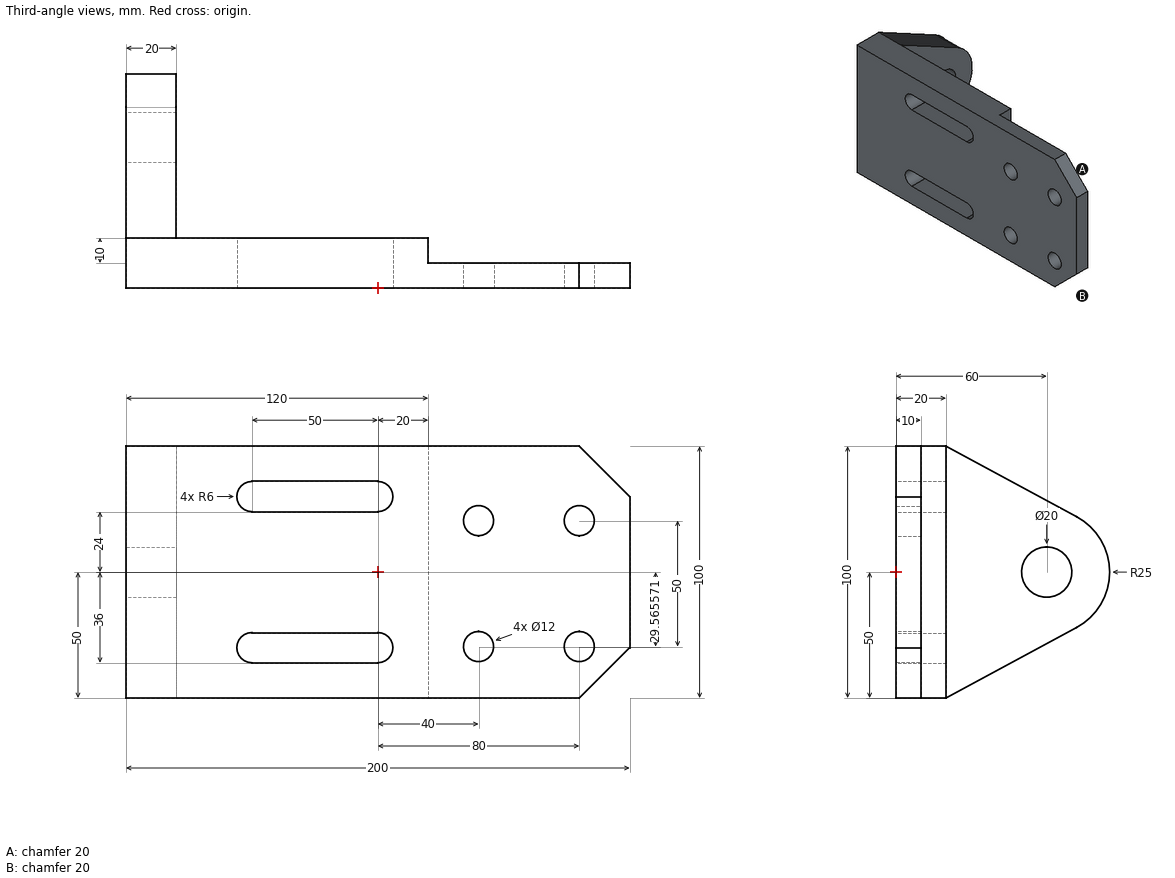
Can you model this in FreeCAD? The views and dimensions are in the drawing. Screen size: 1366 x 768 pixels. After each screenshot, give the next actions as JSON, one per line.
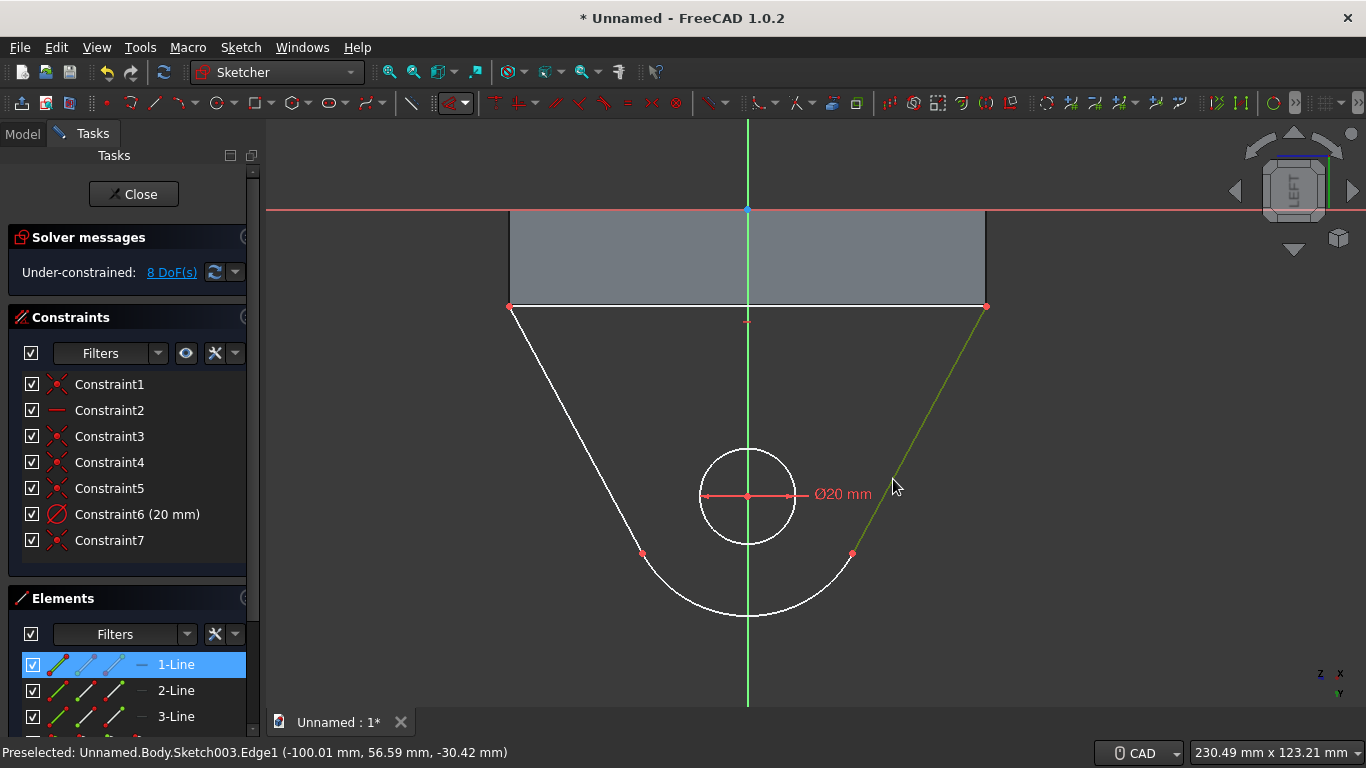
{"action": "left_click", "coordinate": [698, 605]}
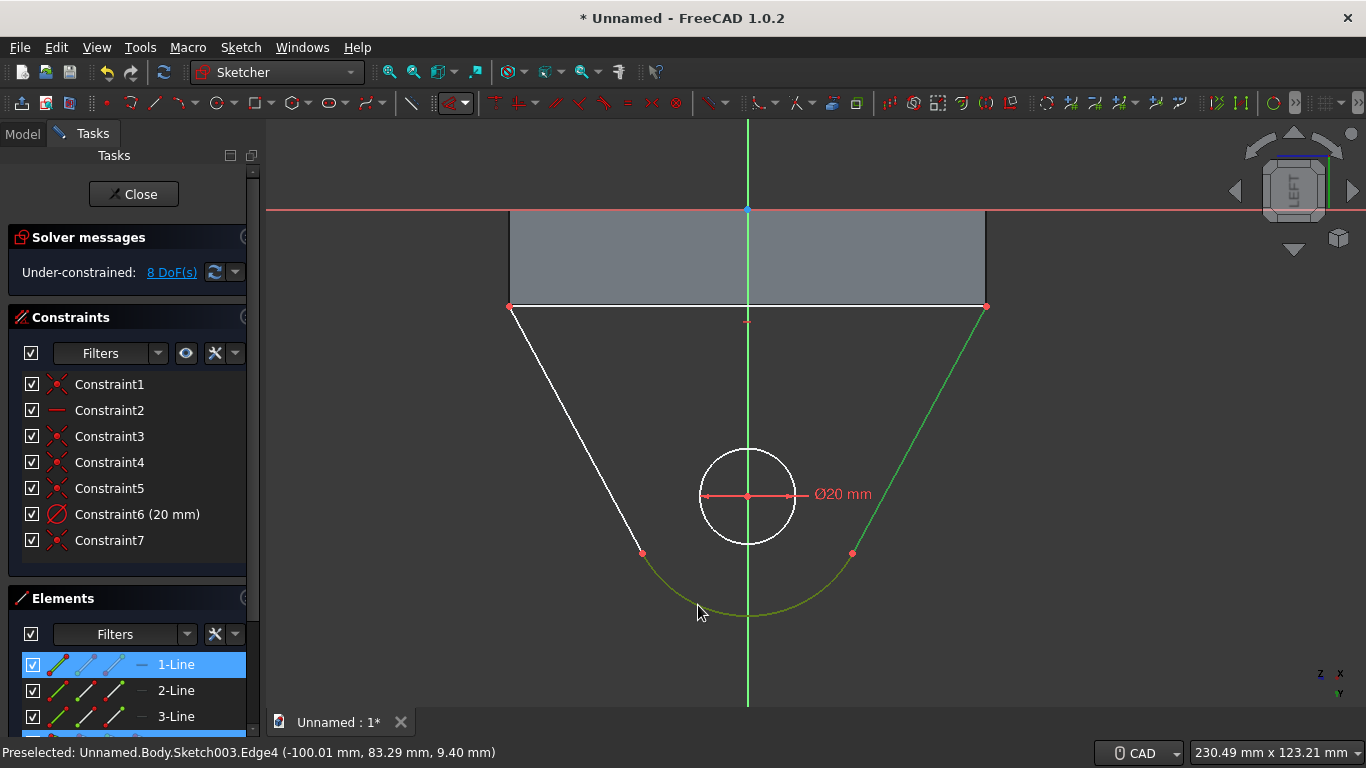
{"action": "left_click", "coordinate": [604, 104]}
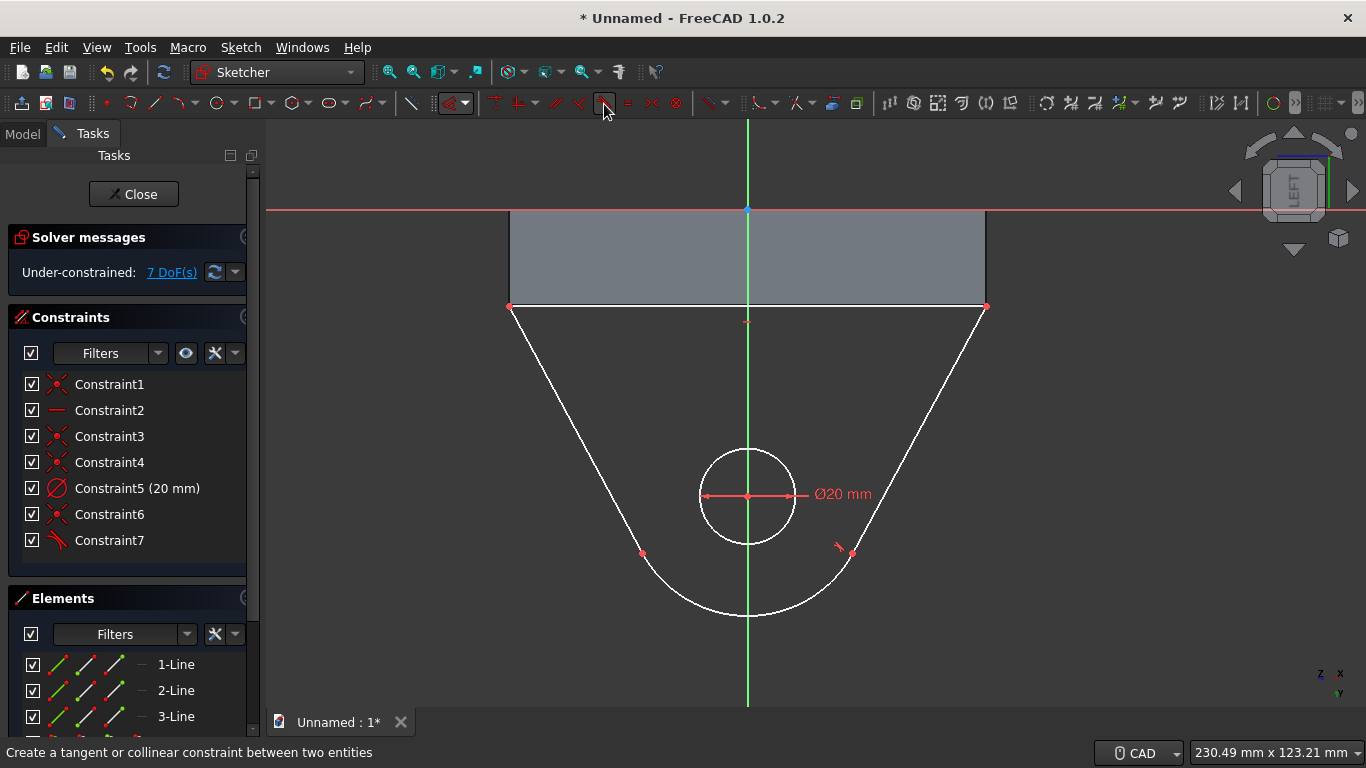
{"action": "left_click", "coordinate": [549, 381]}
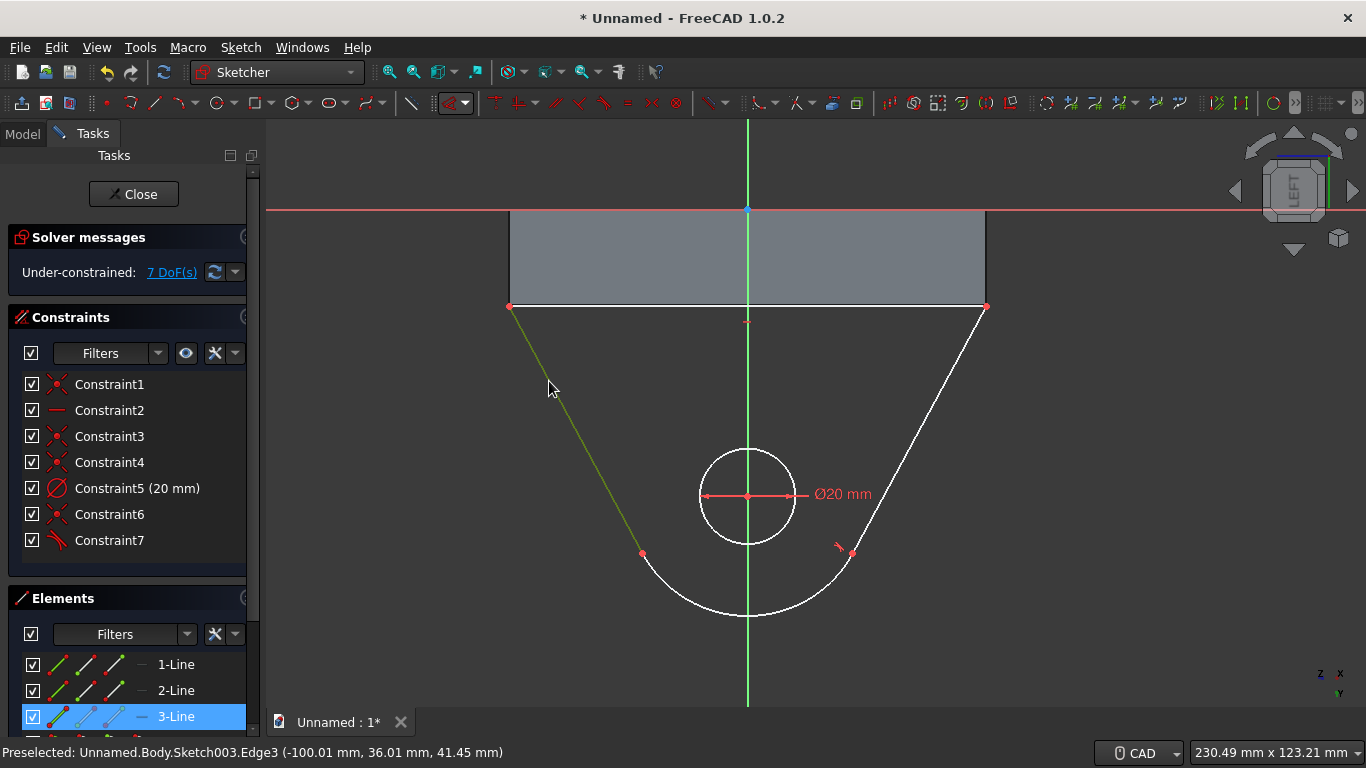
{"action": "left_click", "coordinate": [698, 605]}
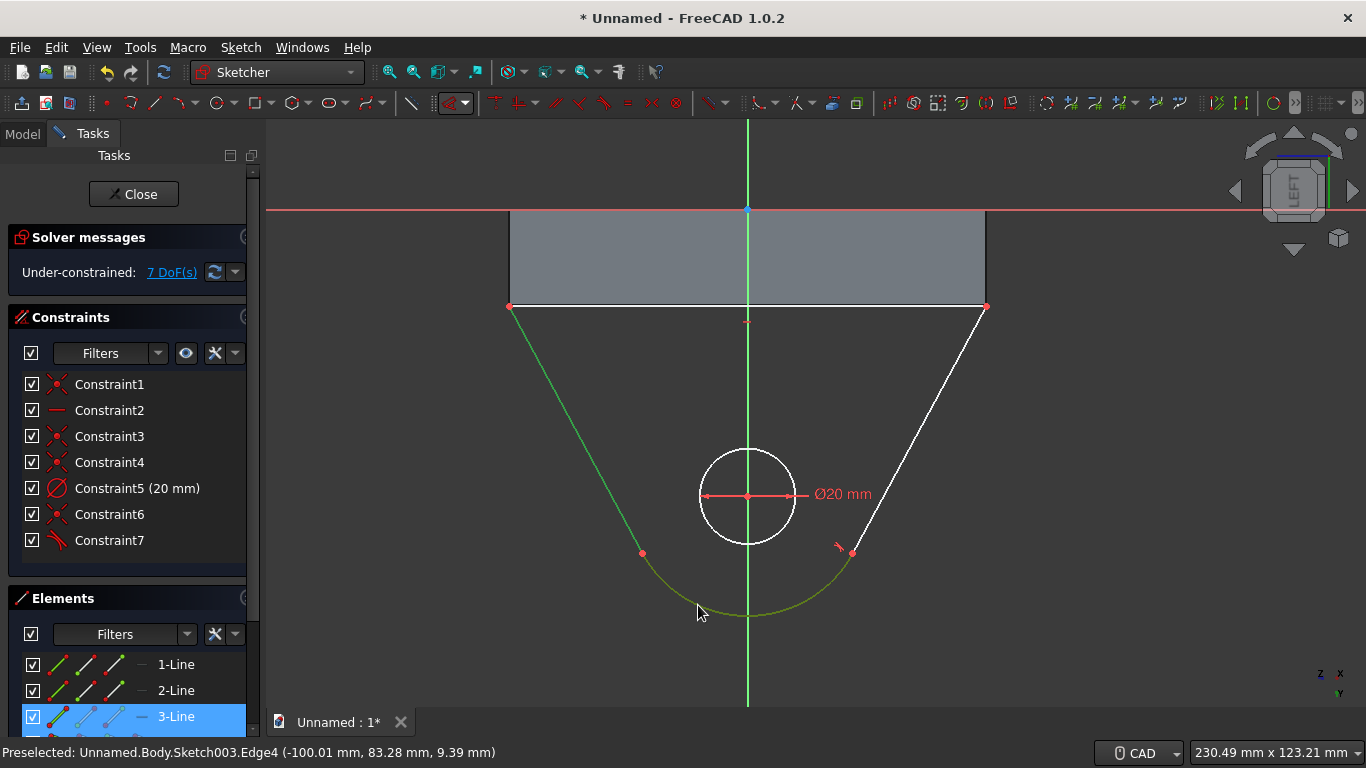
{"action": "left_click", "coordinate": [604, 104]}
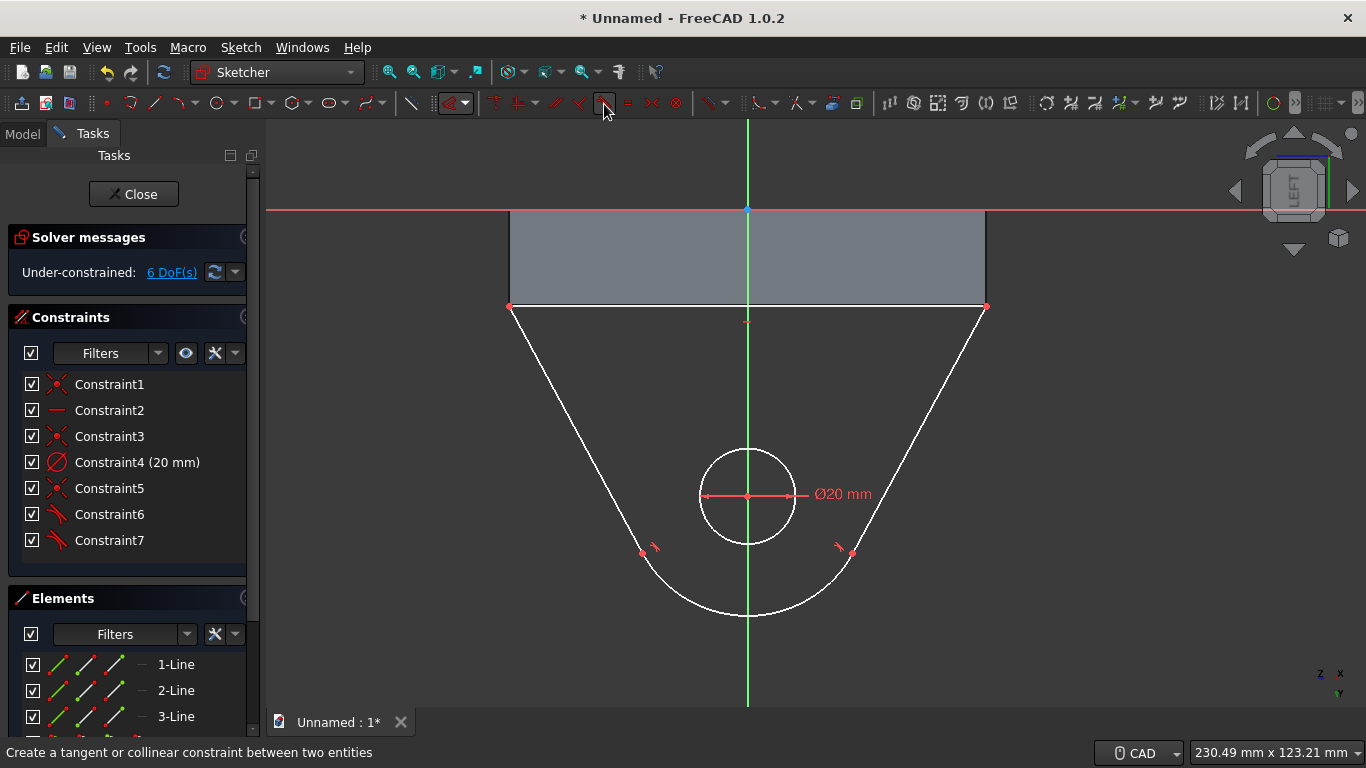
{"action": "left_click", "coordinate": [748, 496]}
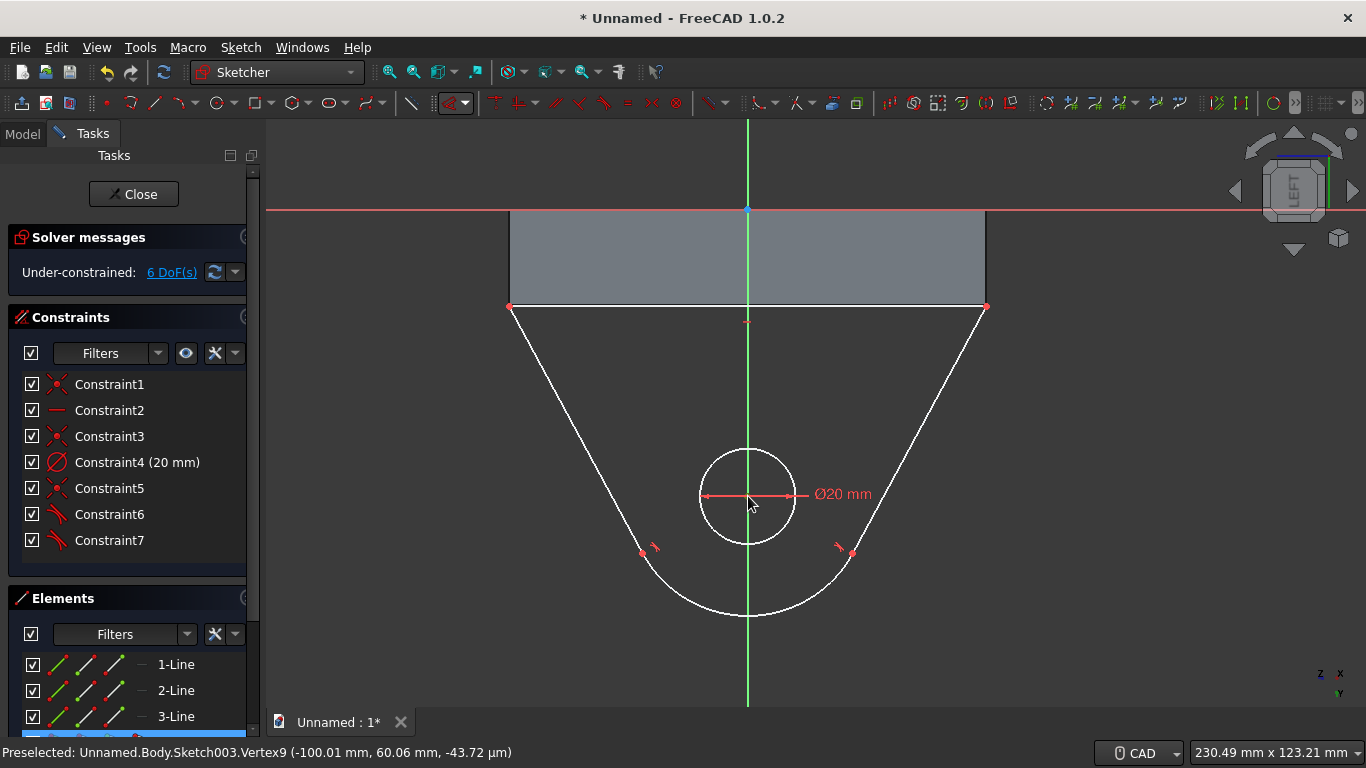
{"action": "left_click", "coordinate": [748, 489]}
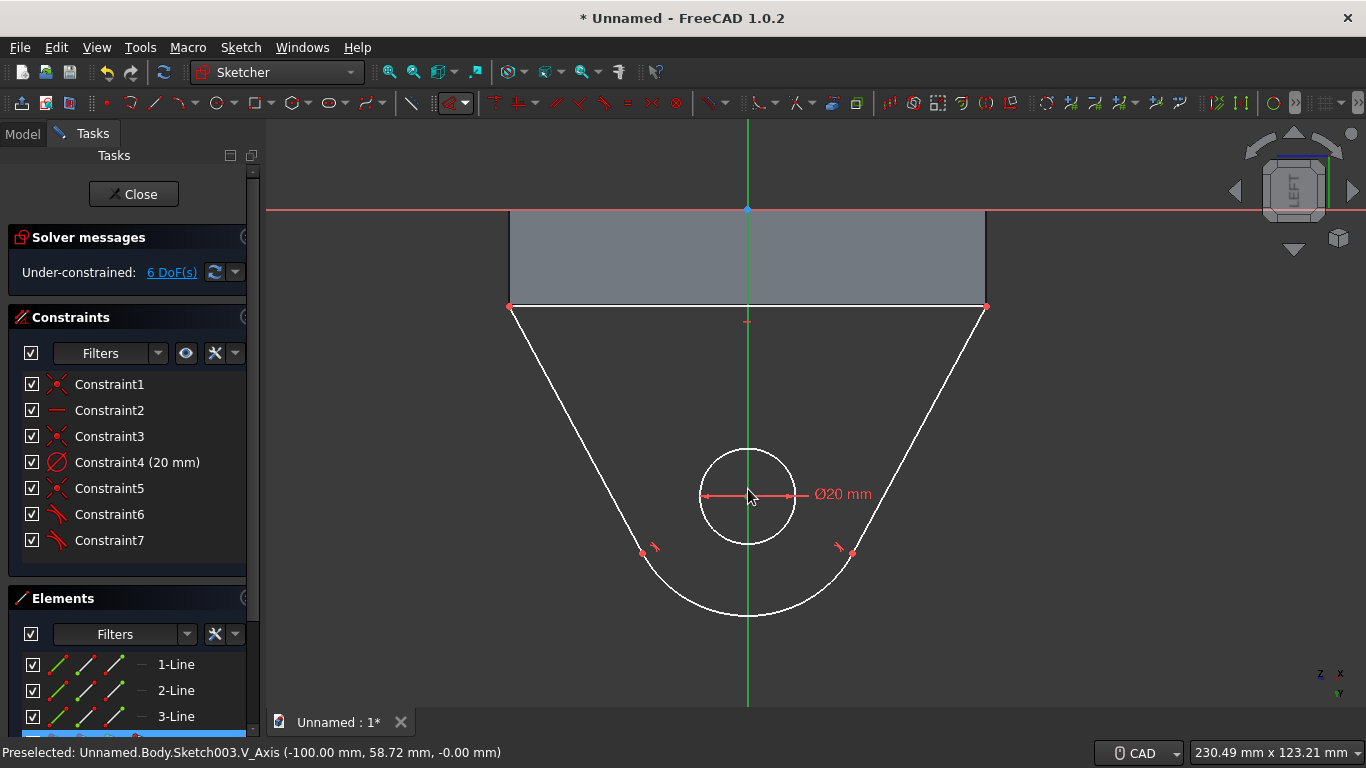
{"action": "left_click", "coordinate": [496, 104]}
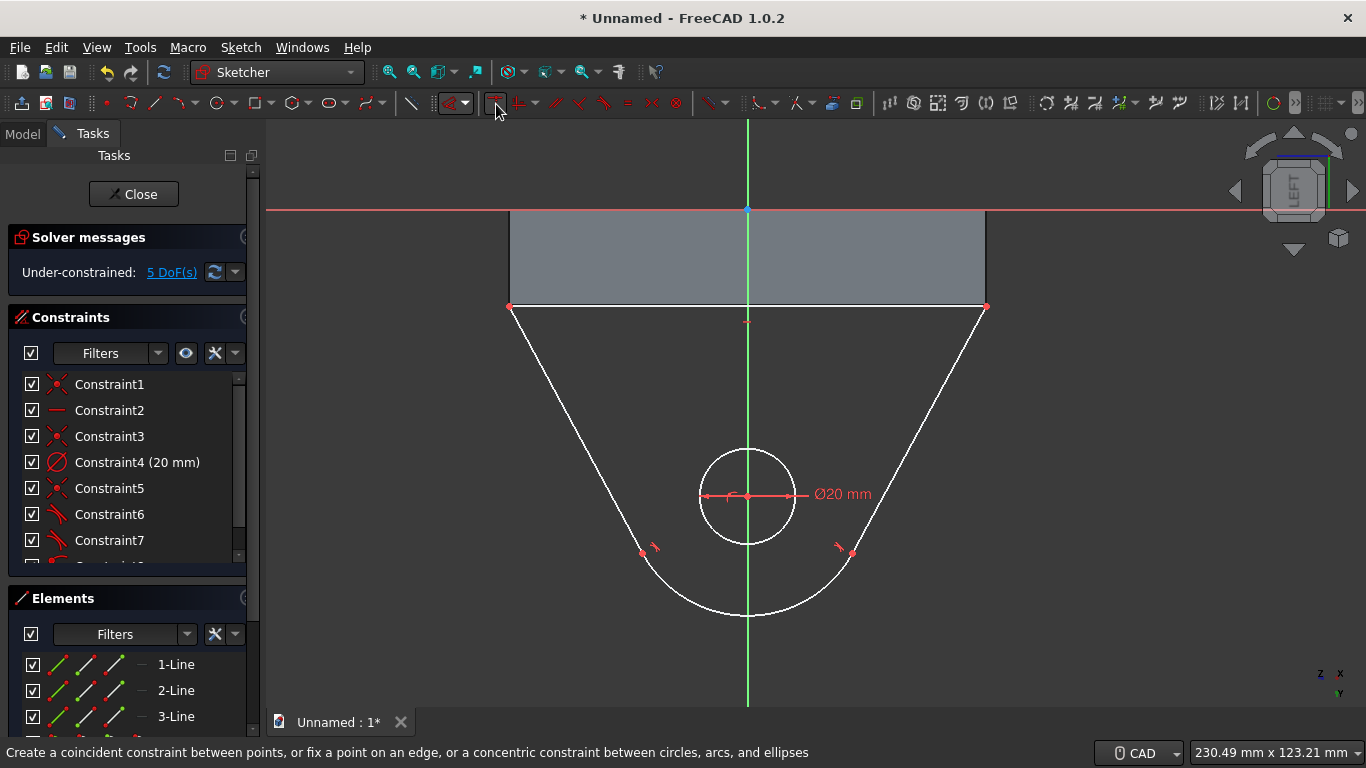
{"action": "left_click", "coordinate": [698, 605]}